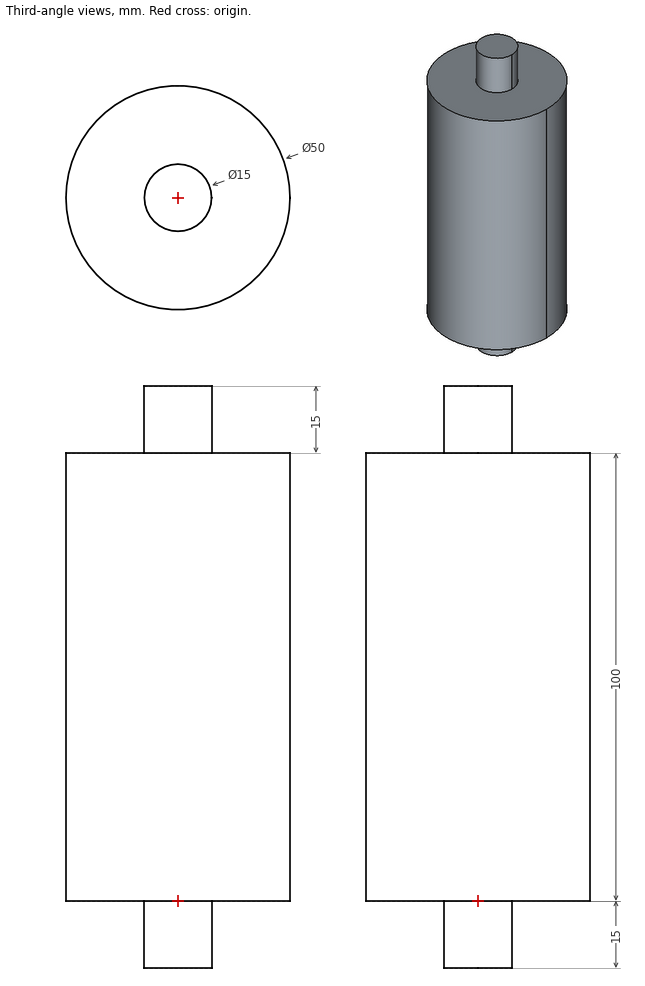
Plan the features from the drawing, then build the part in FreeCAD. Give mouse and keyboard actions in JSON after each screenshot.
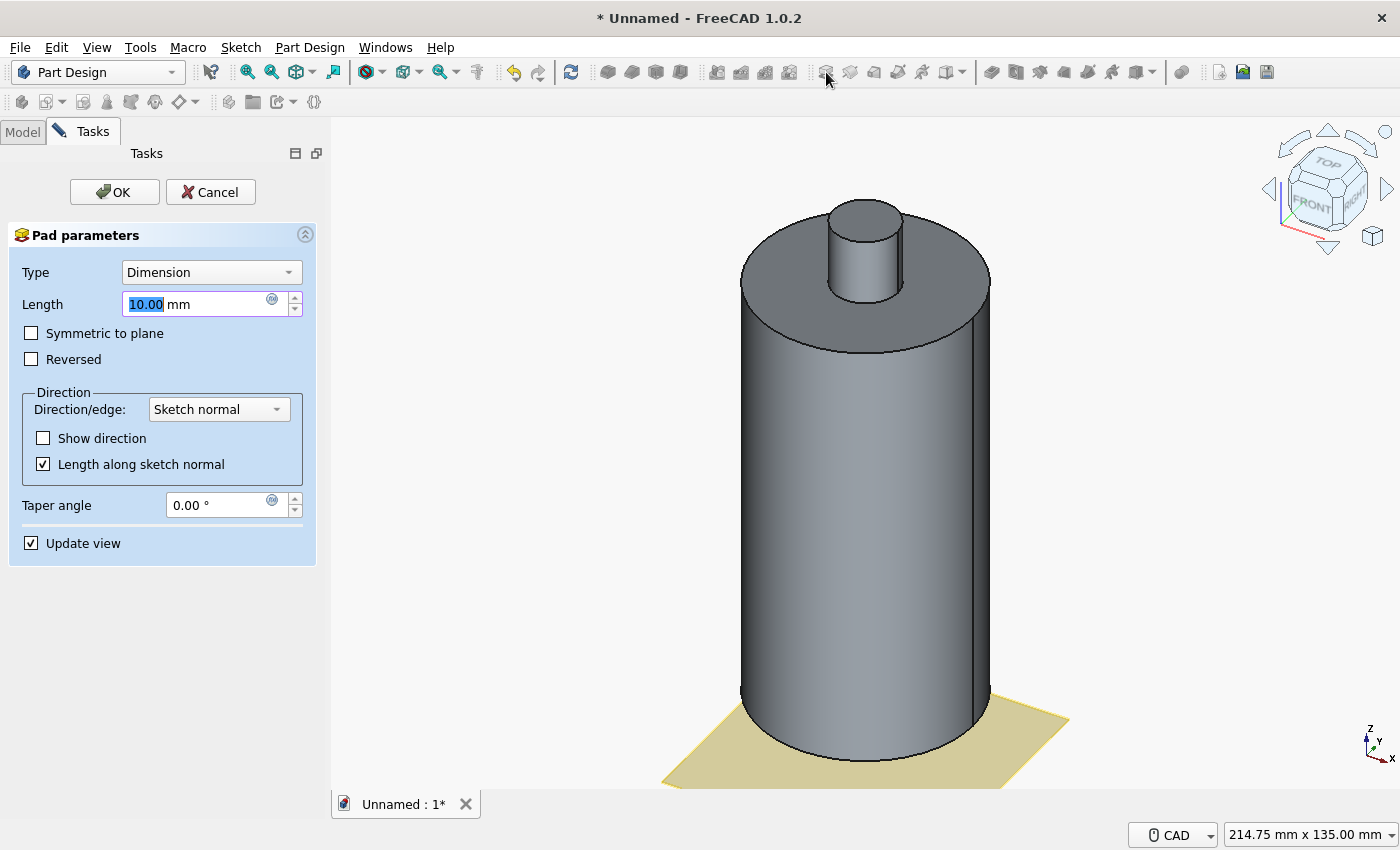
{"action": "type", "text": "15"}
{"action": "key", "text": "Tab"}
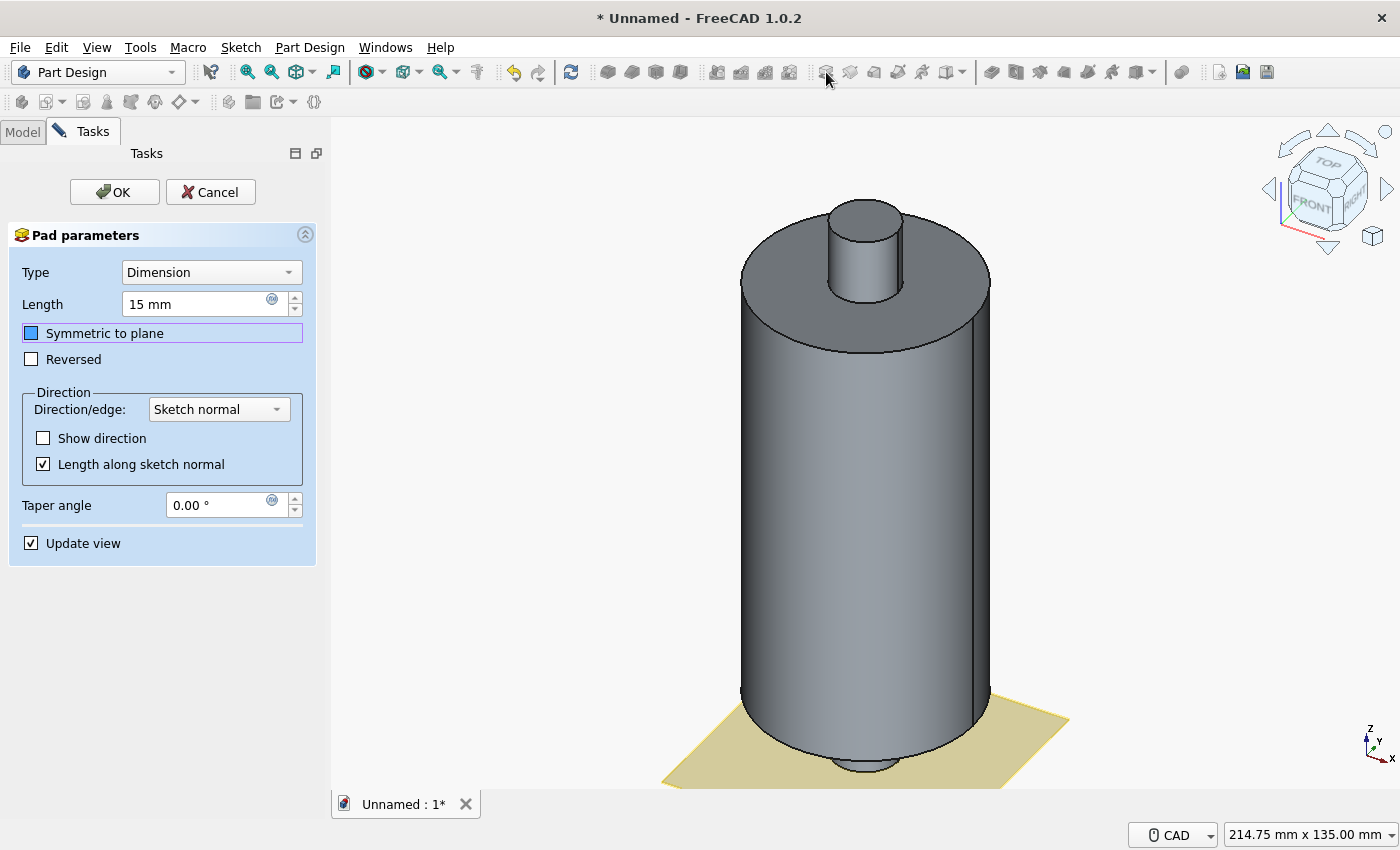
{"action": "left_click", "coordinate": [115, 192]}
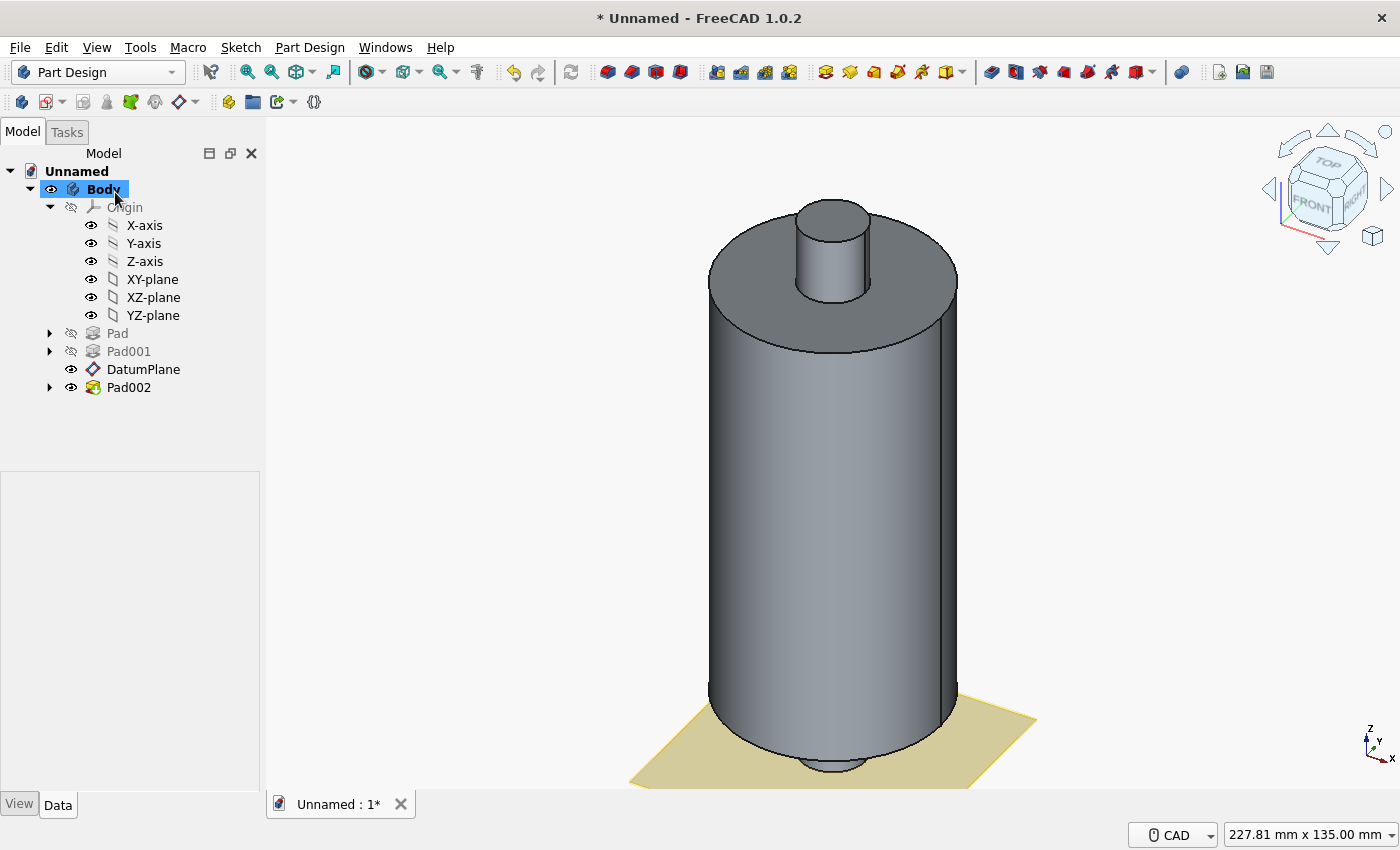
{"action": "left_click", "coordinate": [116, 369]}
{"action": "key", "text": "space"}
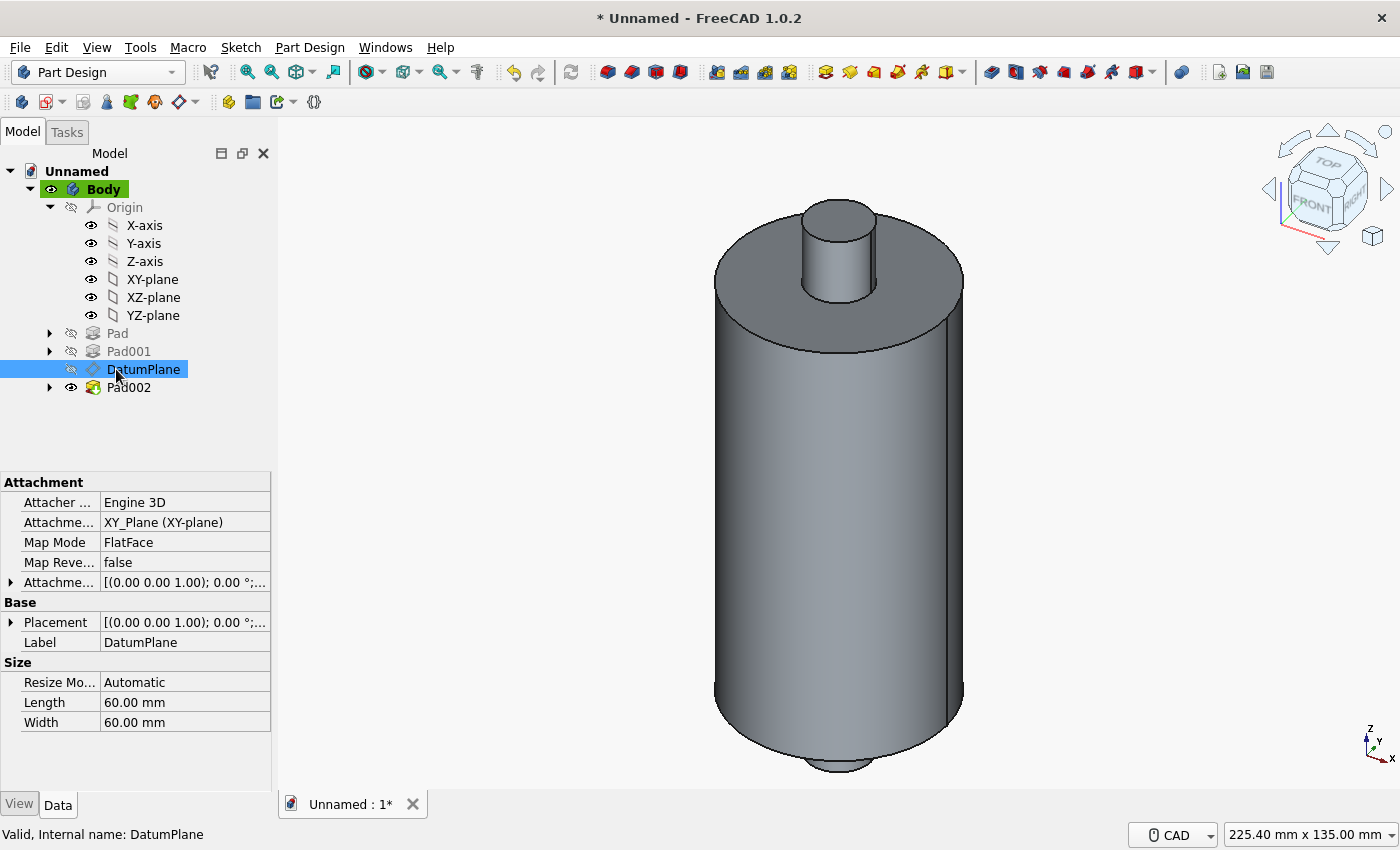
{"action": "key", "text": "0"}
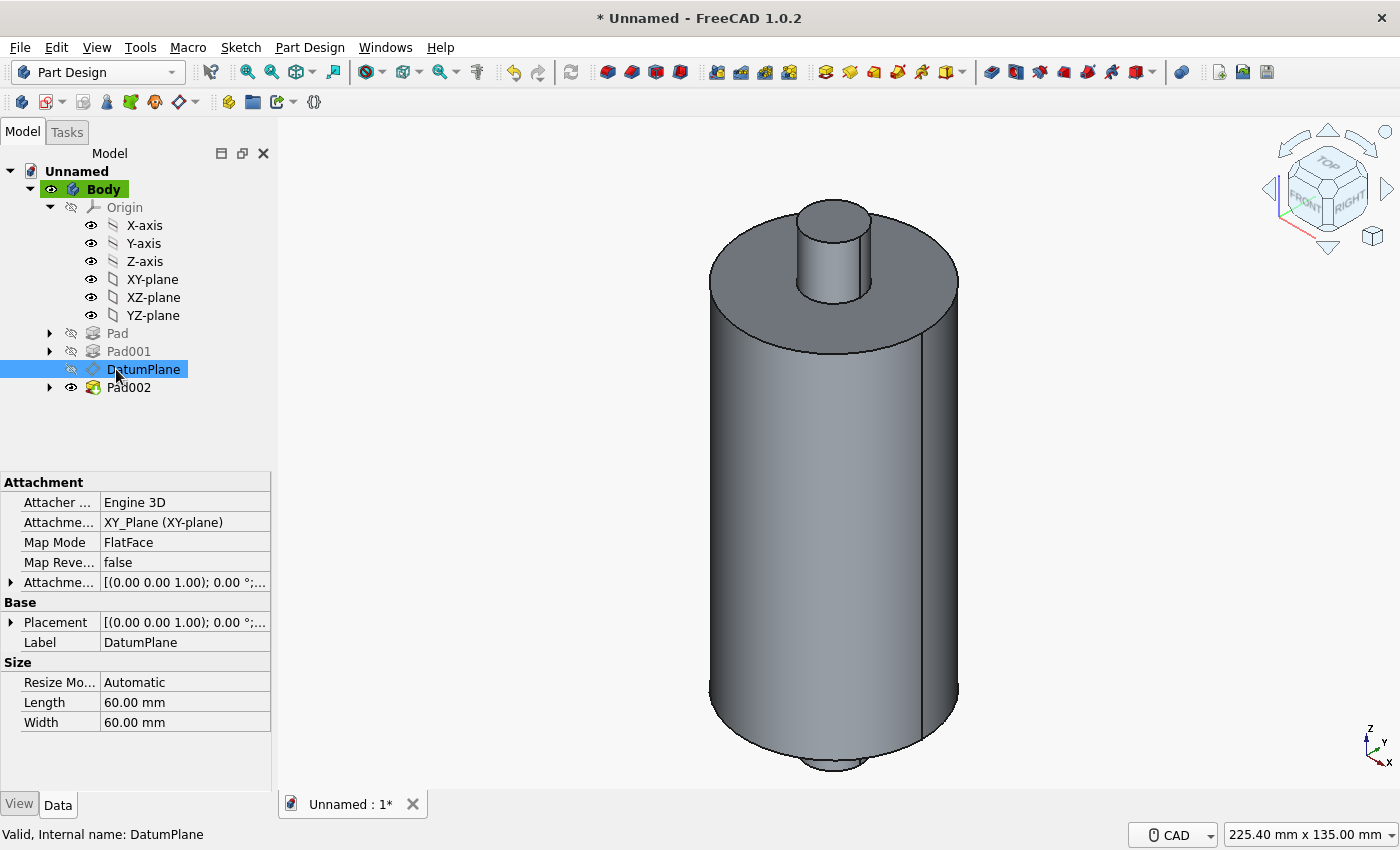
{"action": "left_click", "coordinate": [248, 72]}